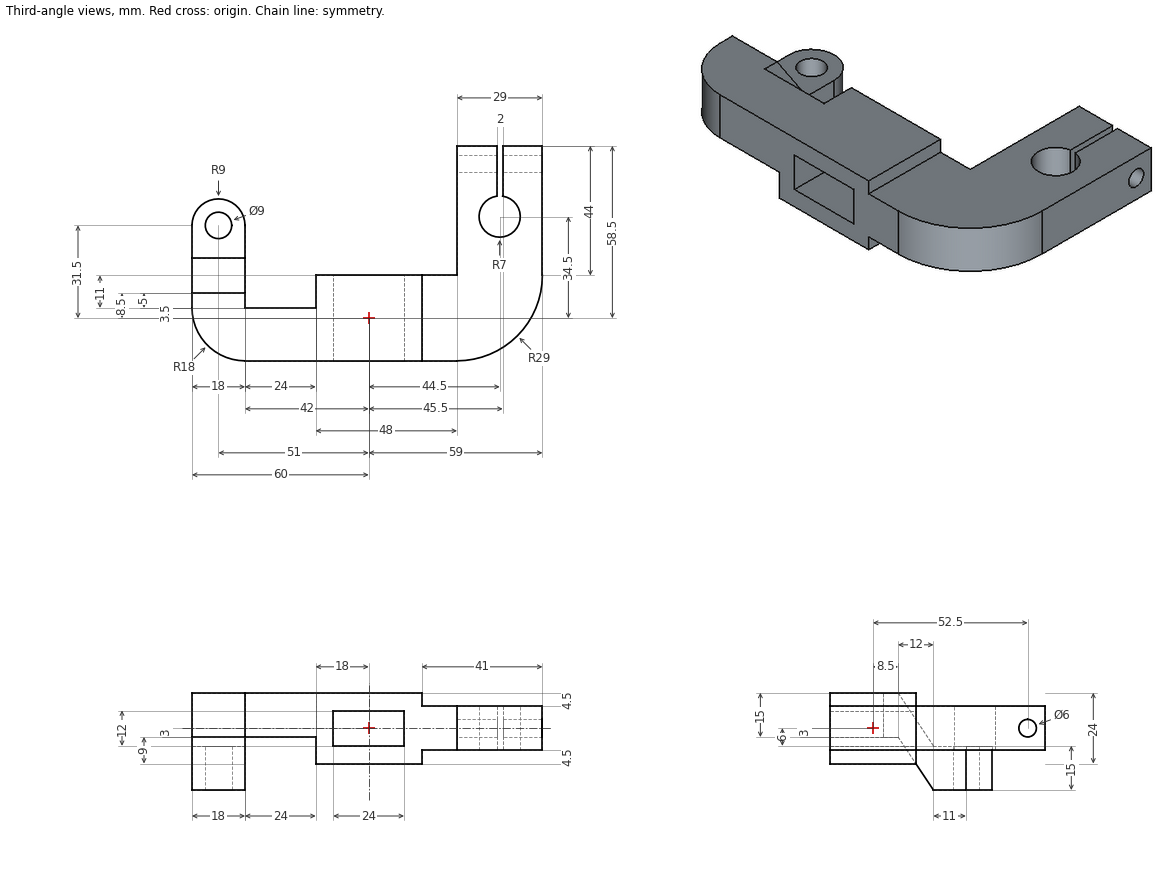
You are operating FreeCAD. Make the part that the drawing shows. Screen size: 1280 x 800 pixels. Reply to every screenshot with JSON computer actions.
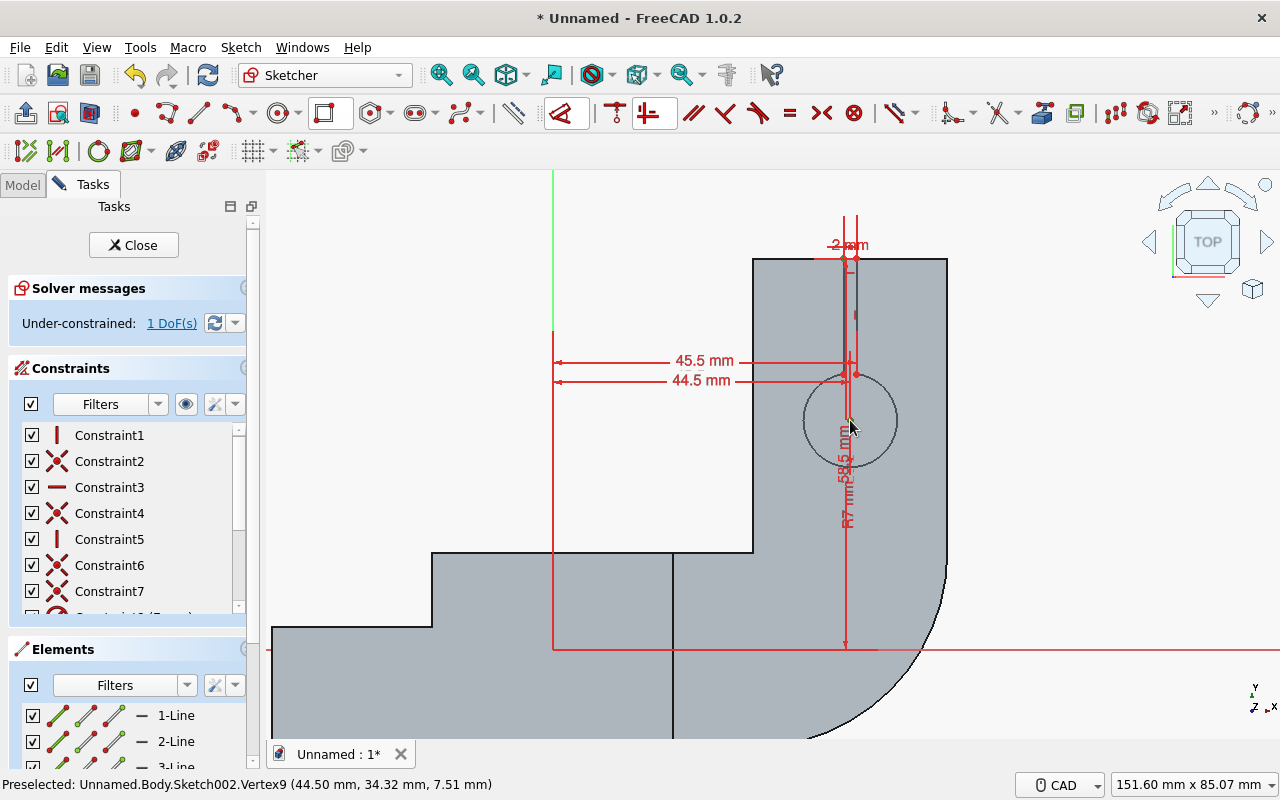
{"action": "left_click", "coordinate": [584, 114]}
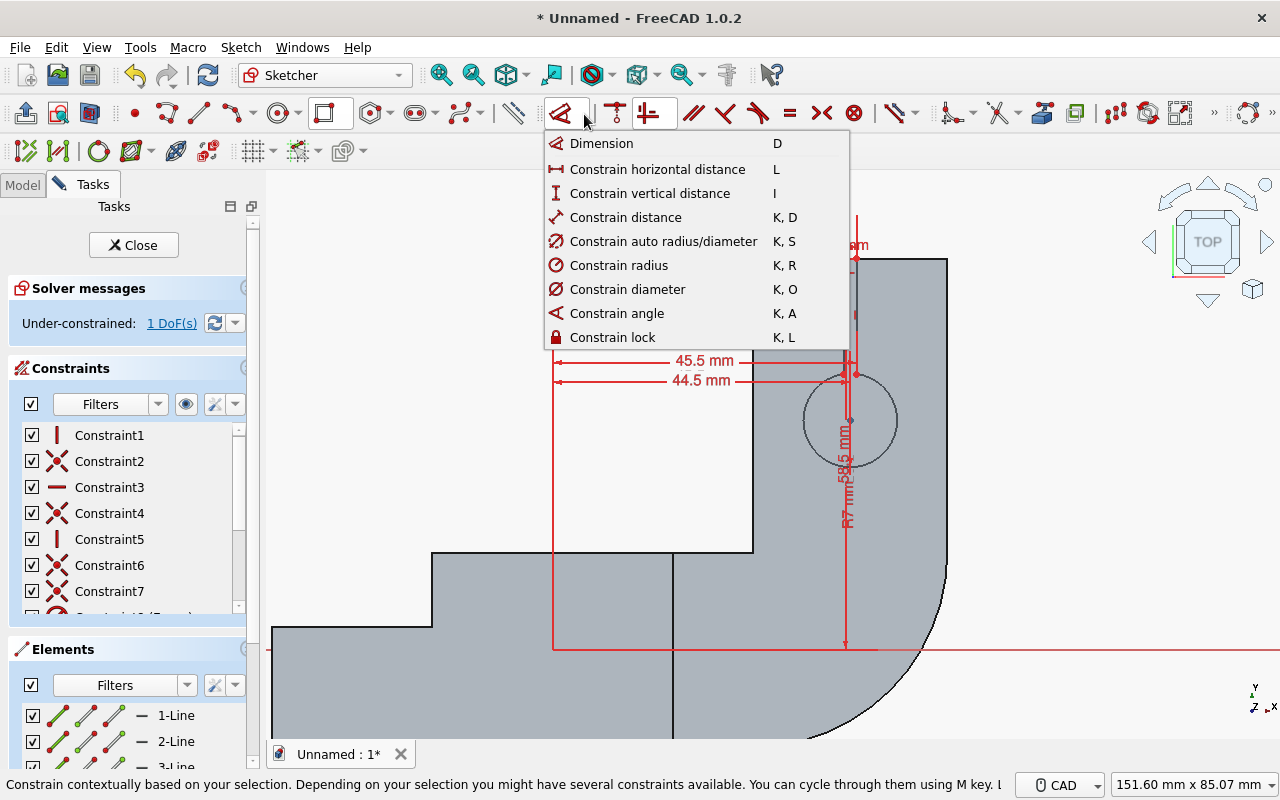
{"action": "left_click", "coordinate": [697, 193]}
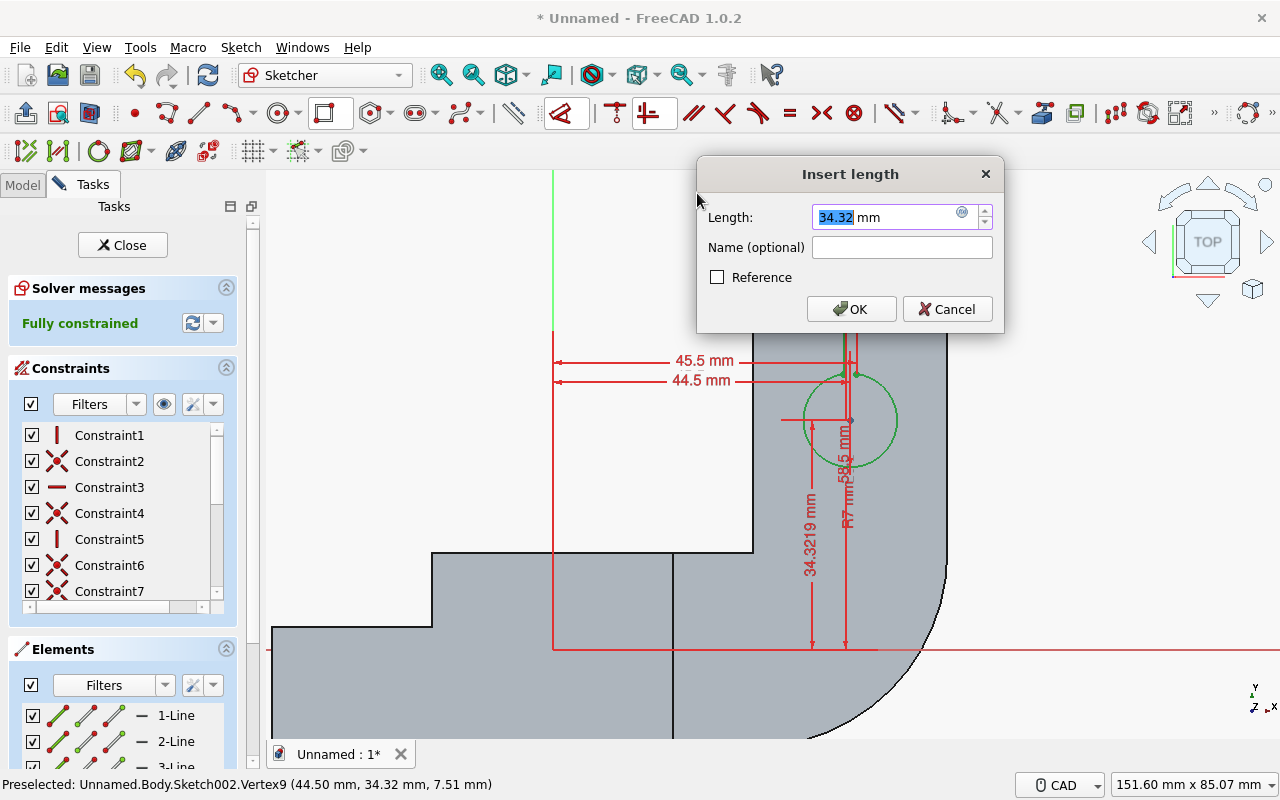
{"action": "type", "text": "34.5"}
{"action": "key", "text": "Return"}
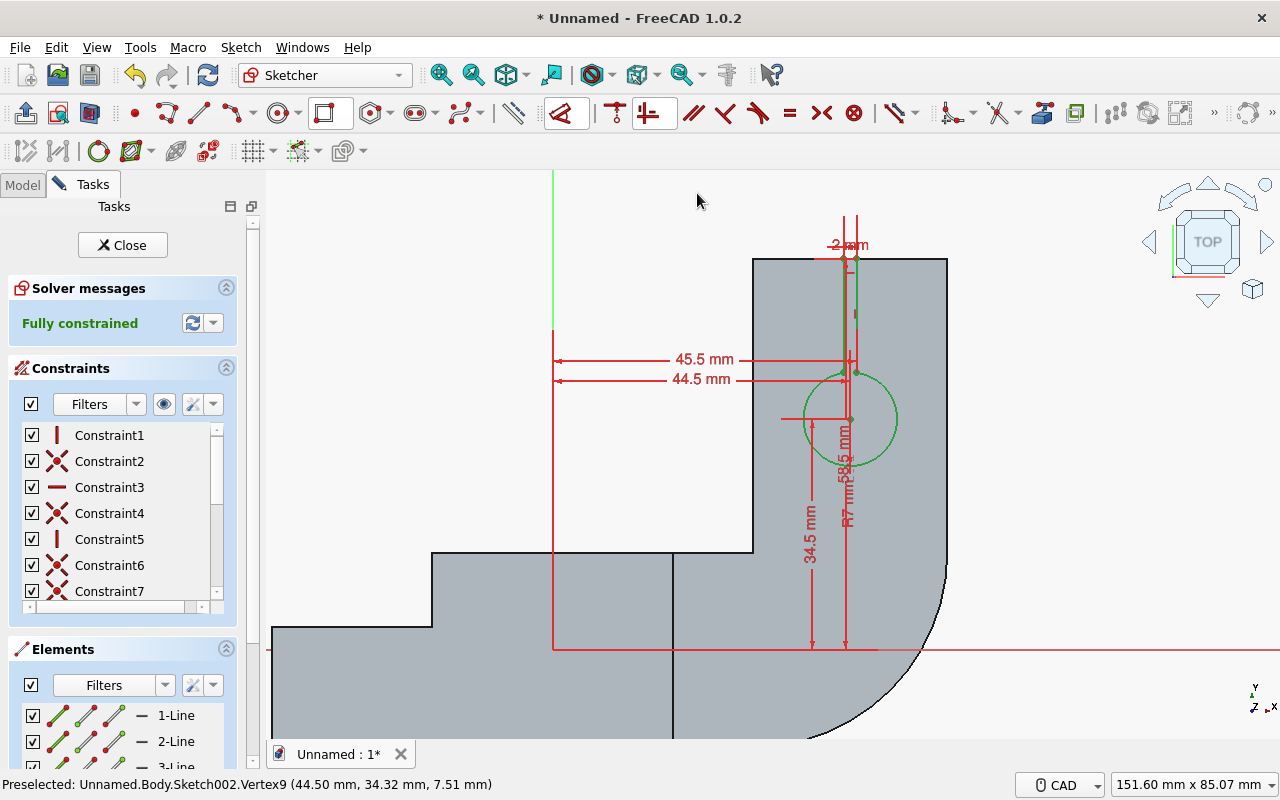
{"action": "left_click", "coordinate": [123, 245]}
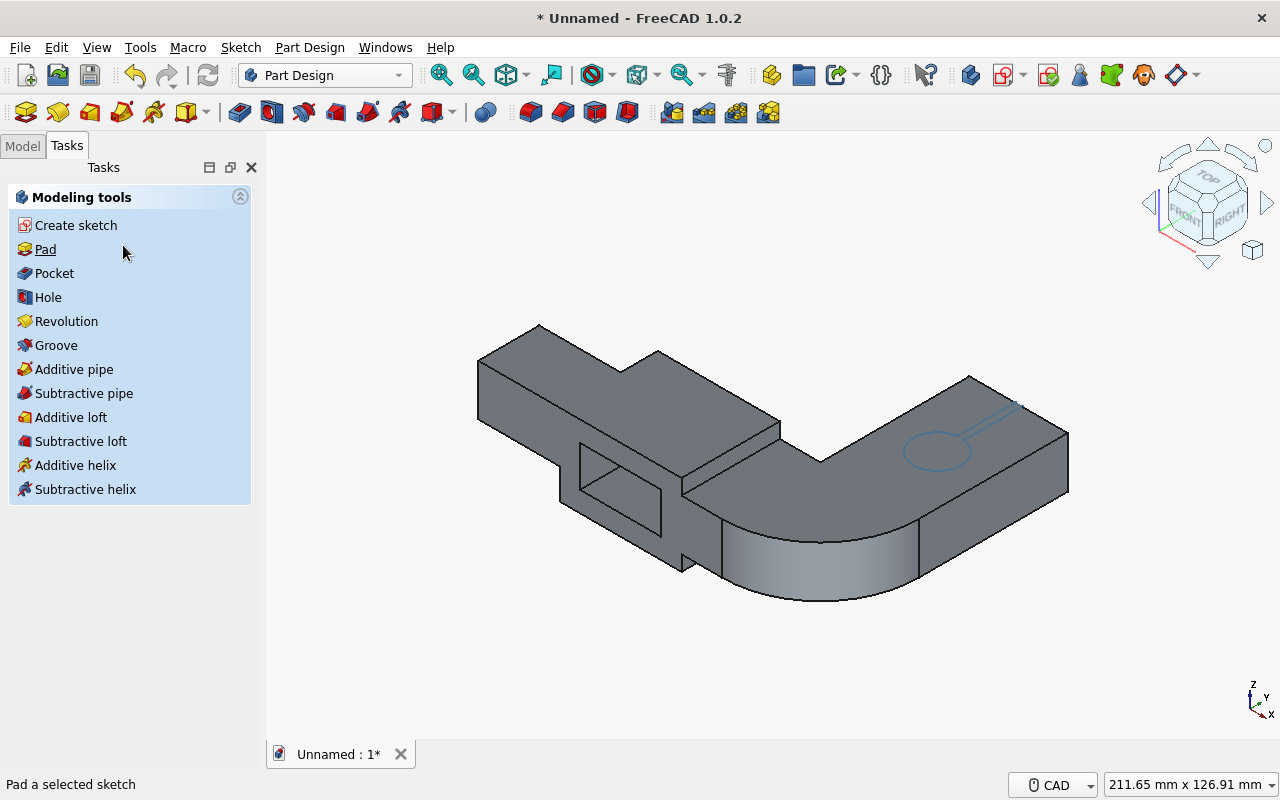
{"action": "left_click", "coordinate": [240, 112]}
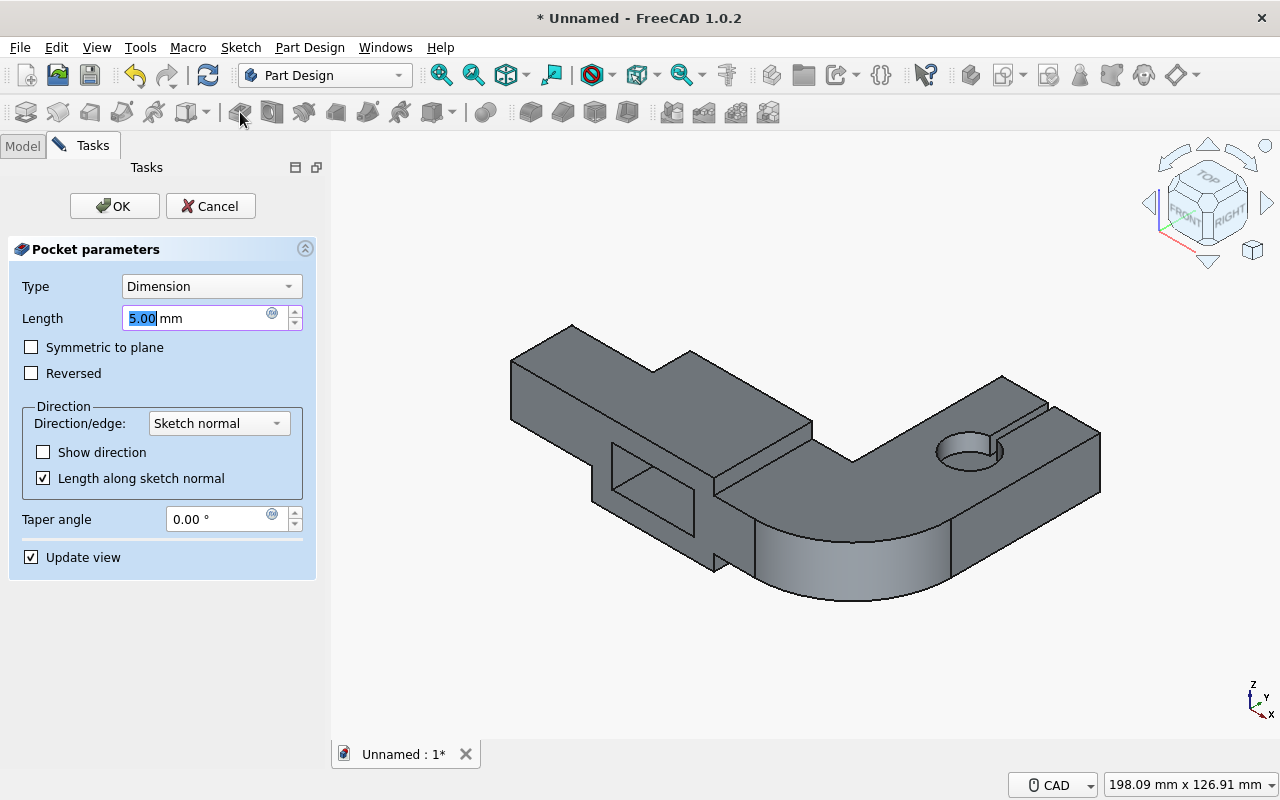
{"action": "left_click", "coordinate": [212, 286]}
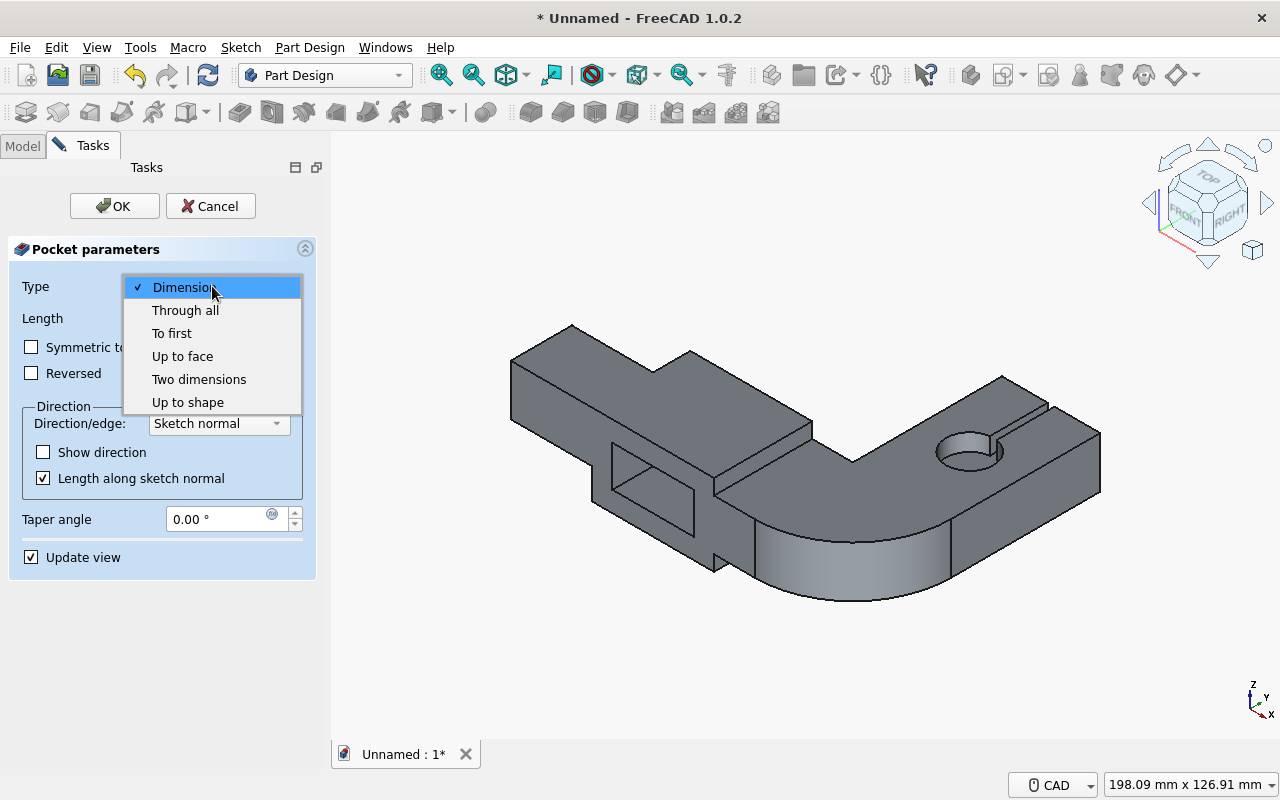
{"action": "left_click", "coordinate": [212, 310]}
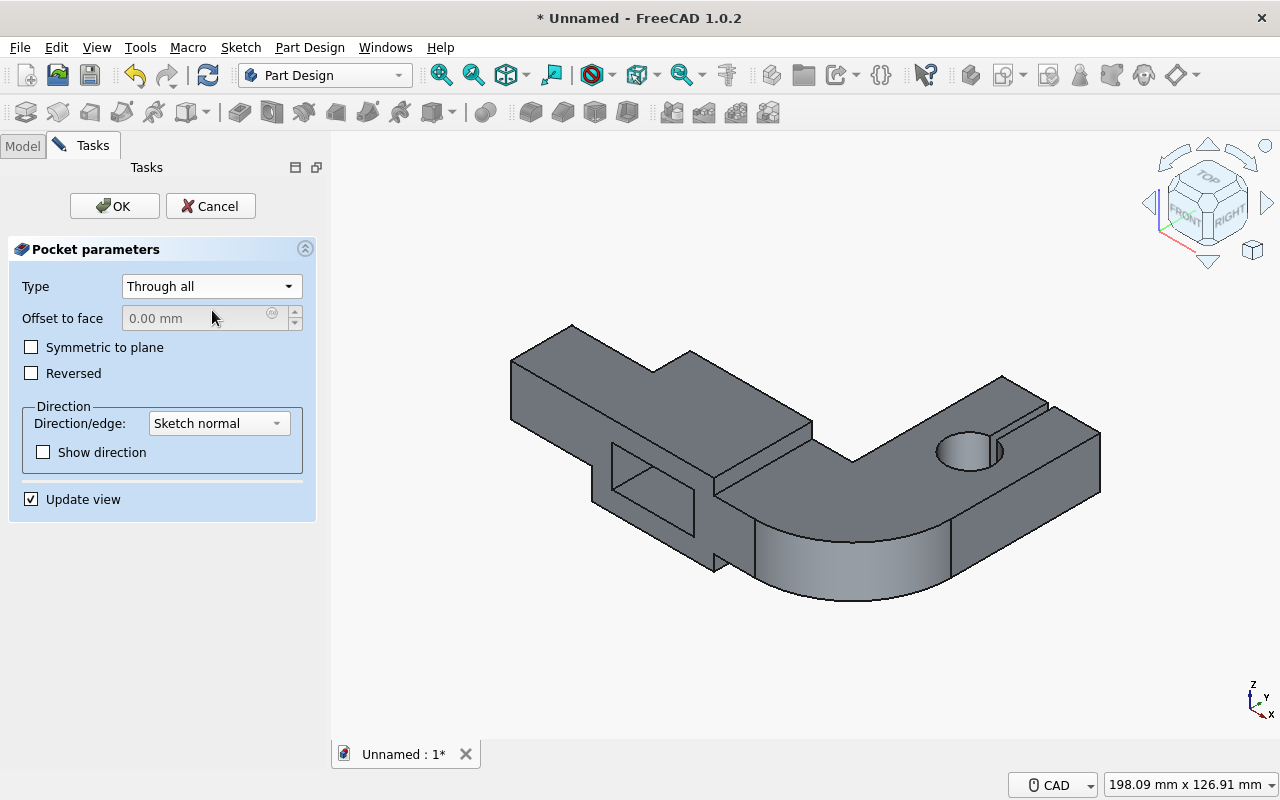
{"action": "left_click", "coordinate": [115, 206]}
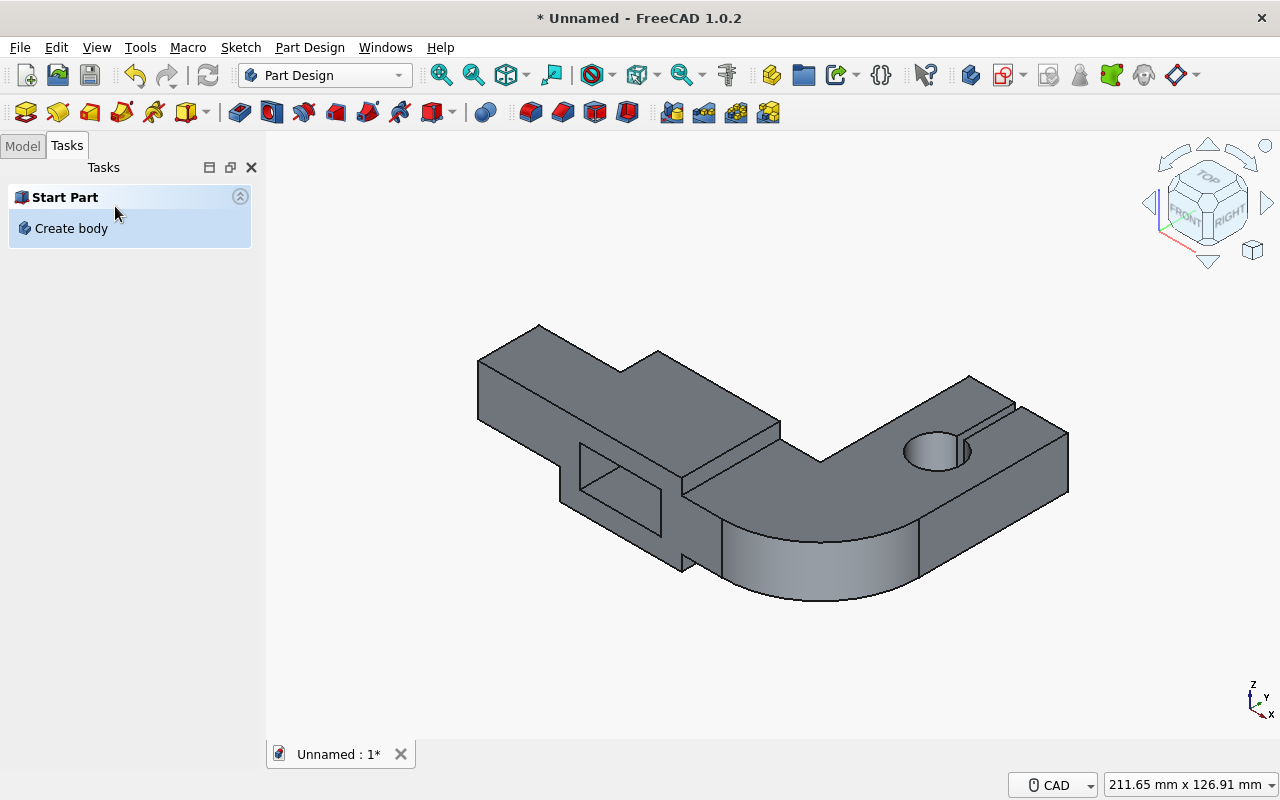
{"action": "key", "text": "6"}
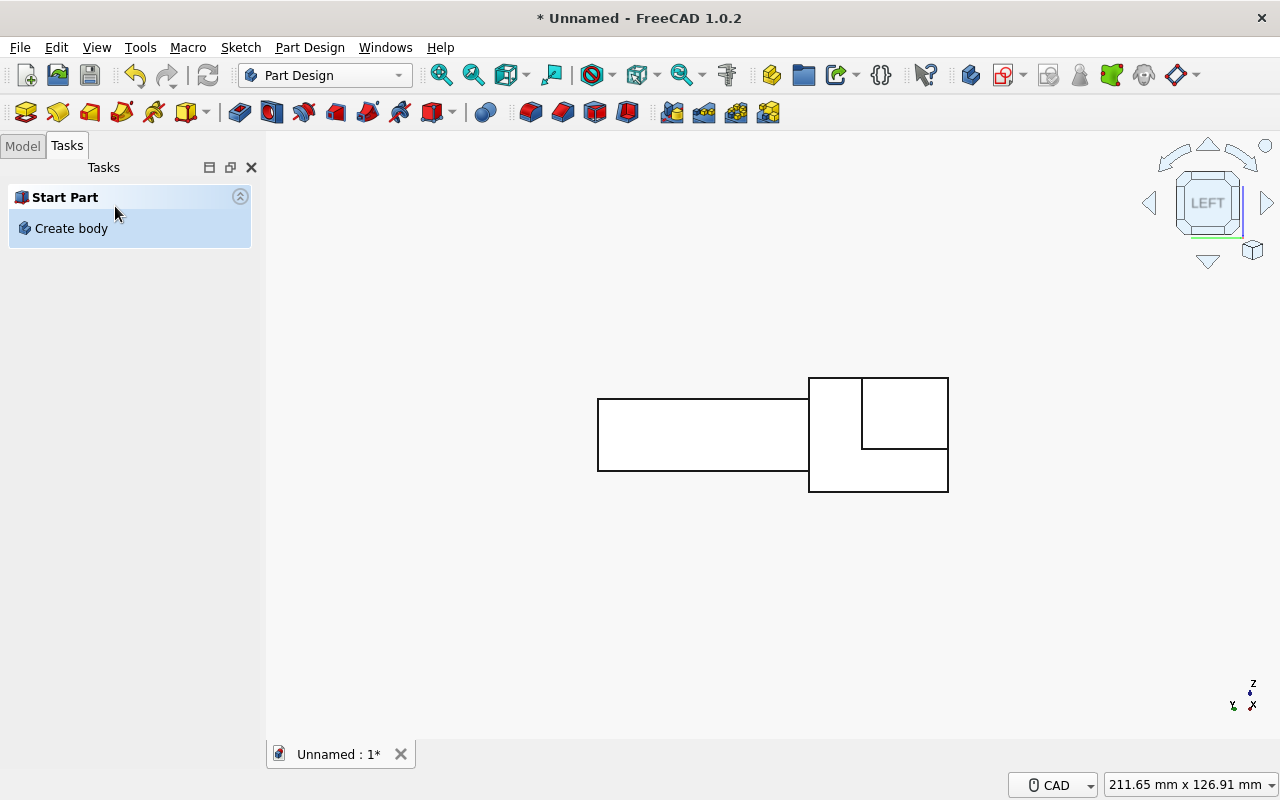
{"action": "left_click", "coordinate": [442, 76]}